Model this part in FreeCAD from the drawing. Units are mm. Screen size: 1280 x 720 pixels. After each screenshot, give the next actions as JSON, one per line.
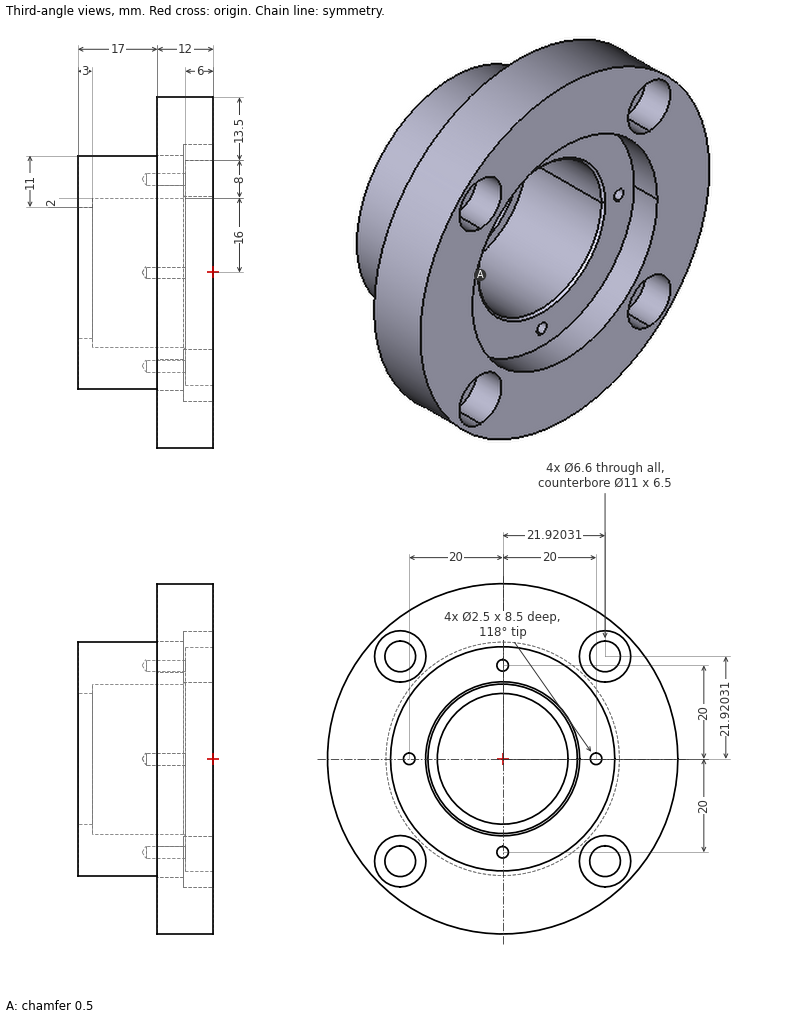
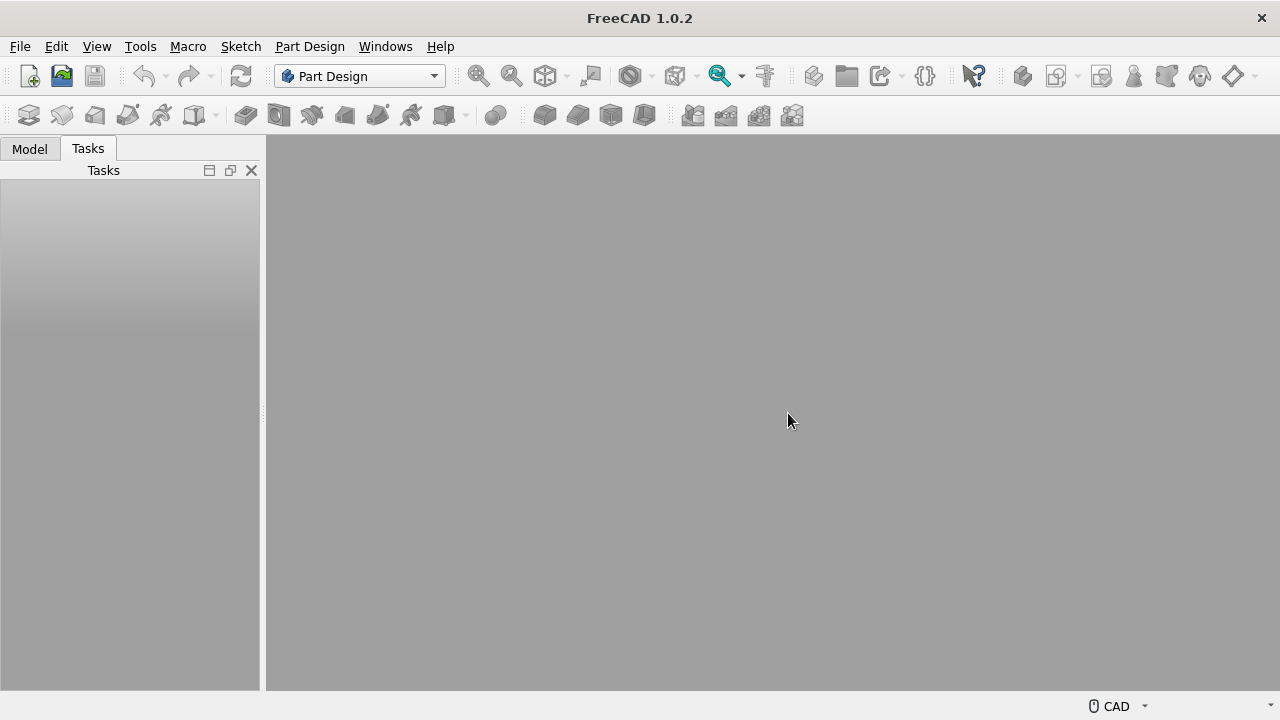
{"action": "key", "text": "ctrl+n"}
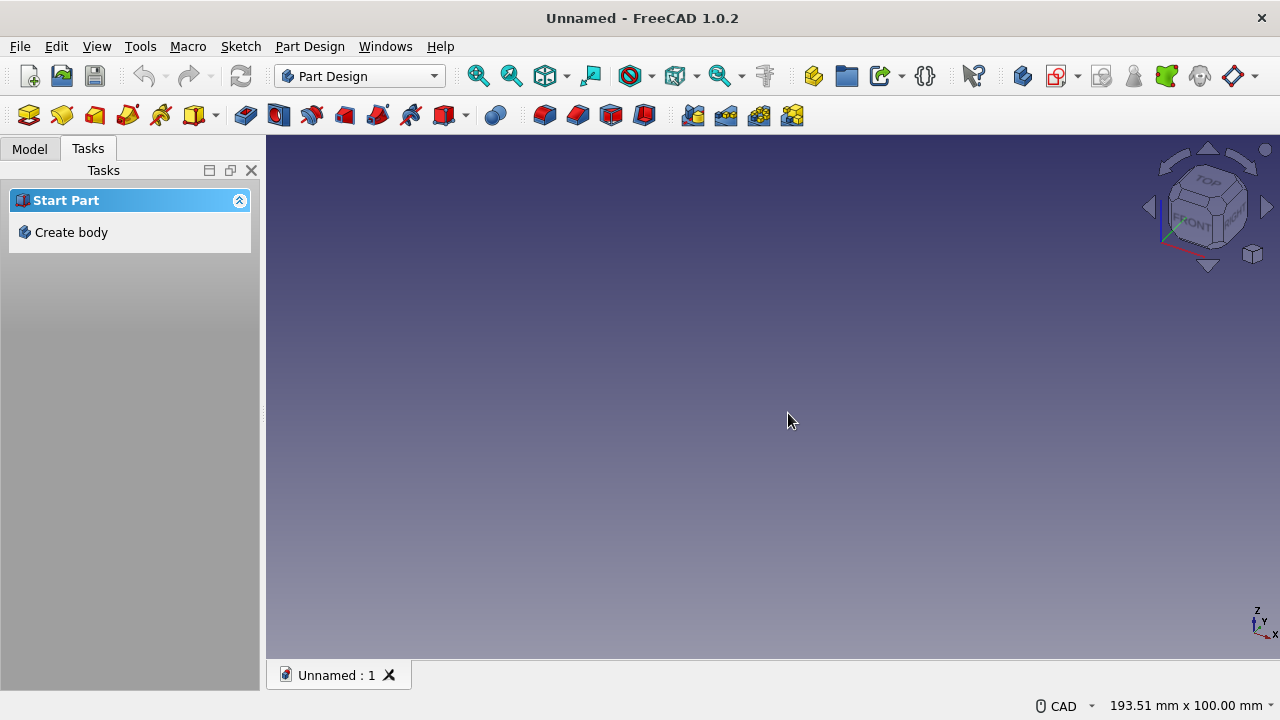
{"action": "left_click", "coordinate": [1056, 76]}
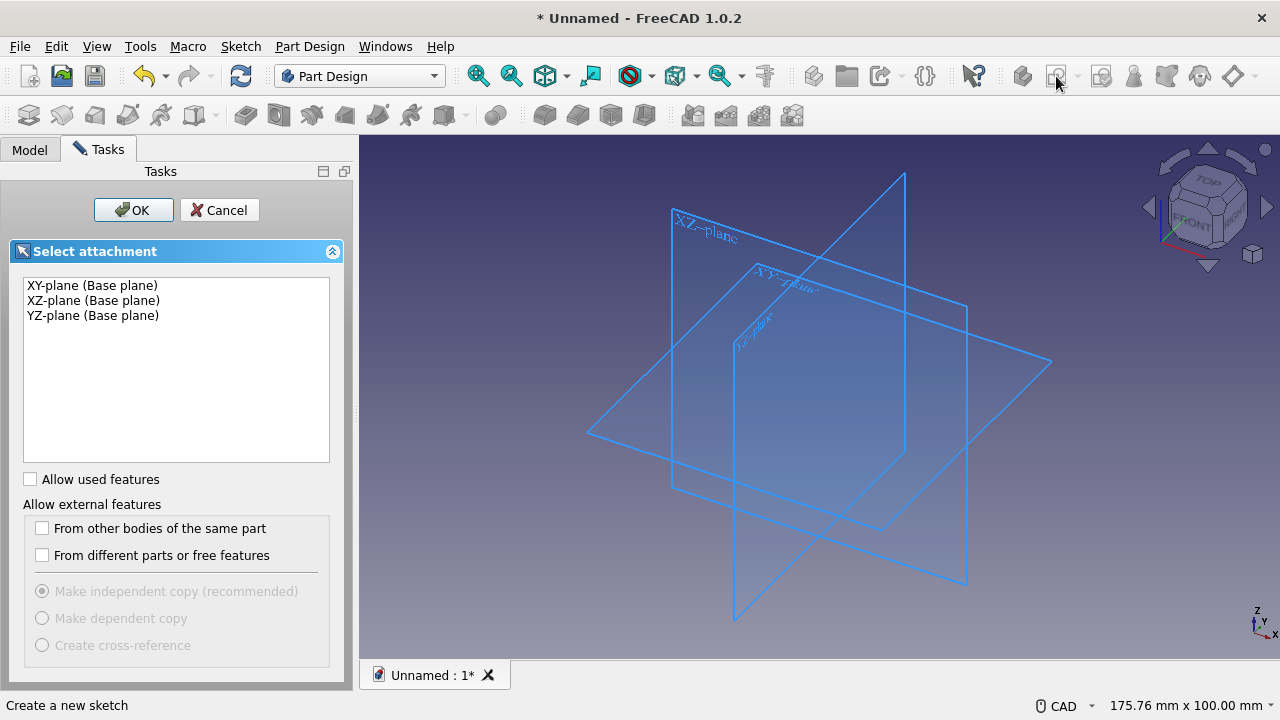
{"action": "left_click", "coordinate": [84, 286]}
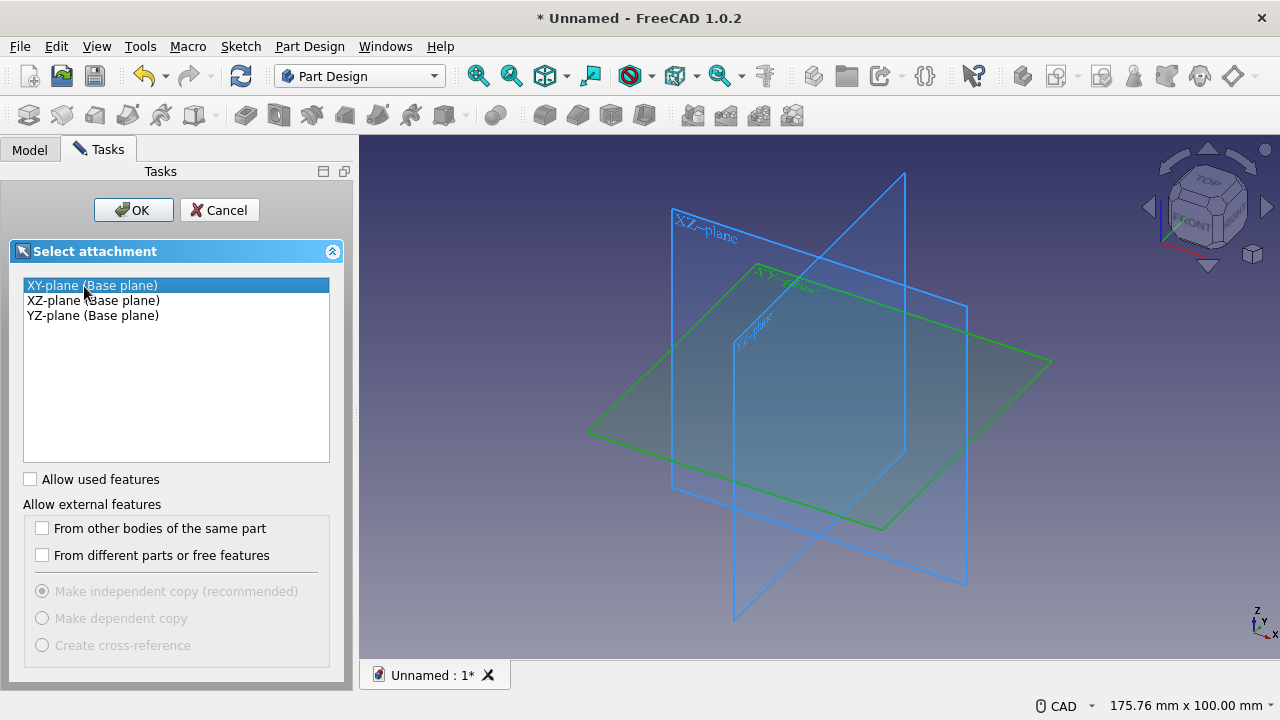
{"action": "left_click", "coordinate": [134, 210]}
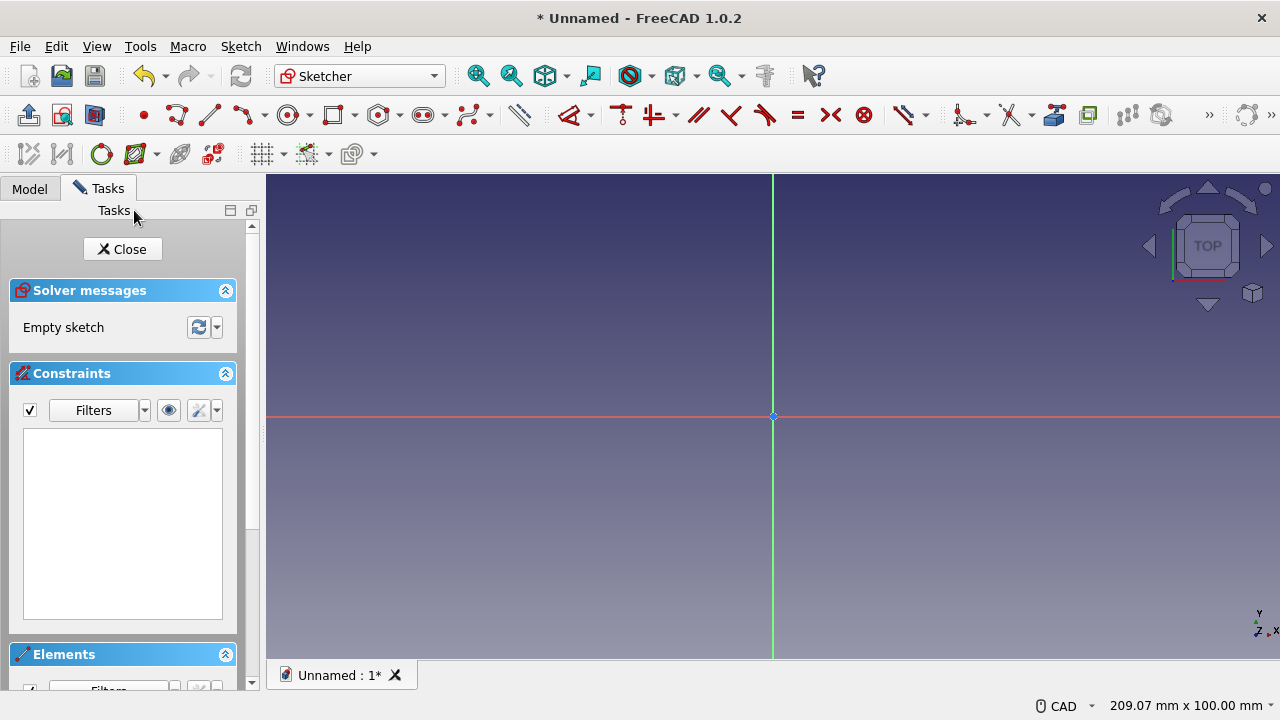
{"action": "scroll", "coordinate": [700, 215], "scroll_direction": "up", "scroll_amount": 3}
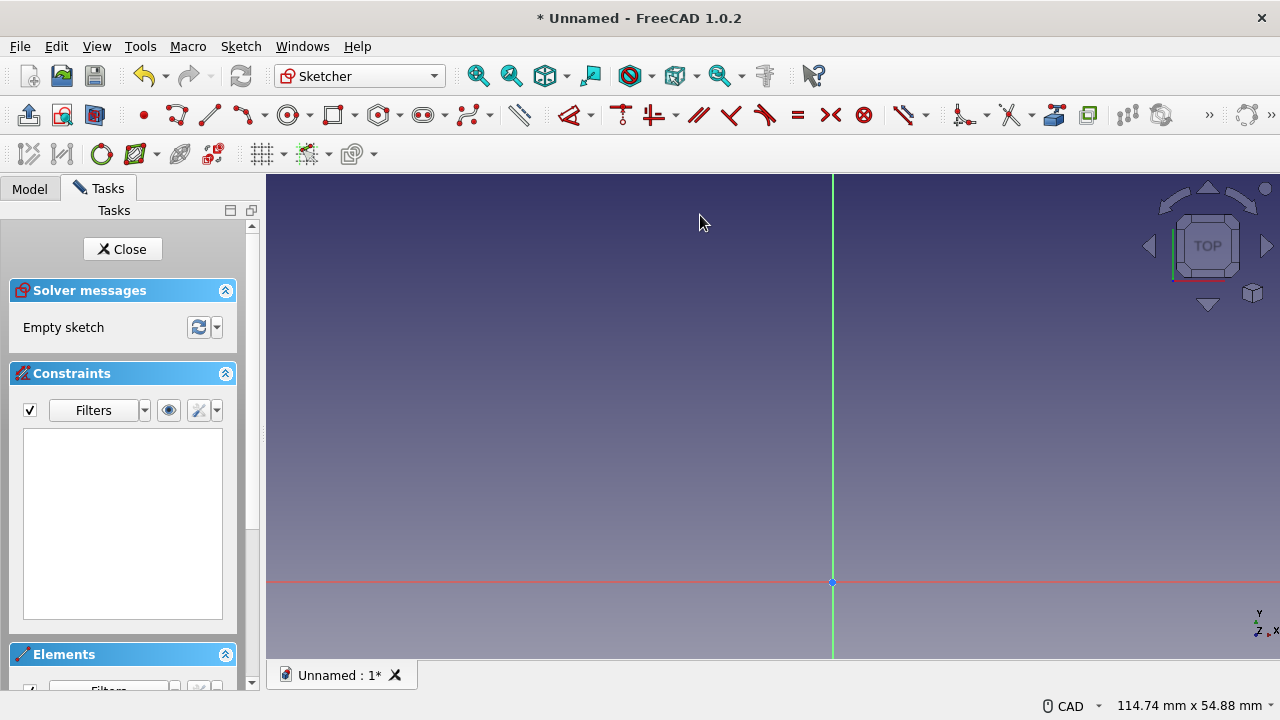
{"action": "key", "text": "g m"}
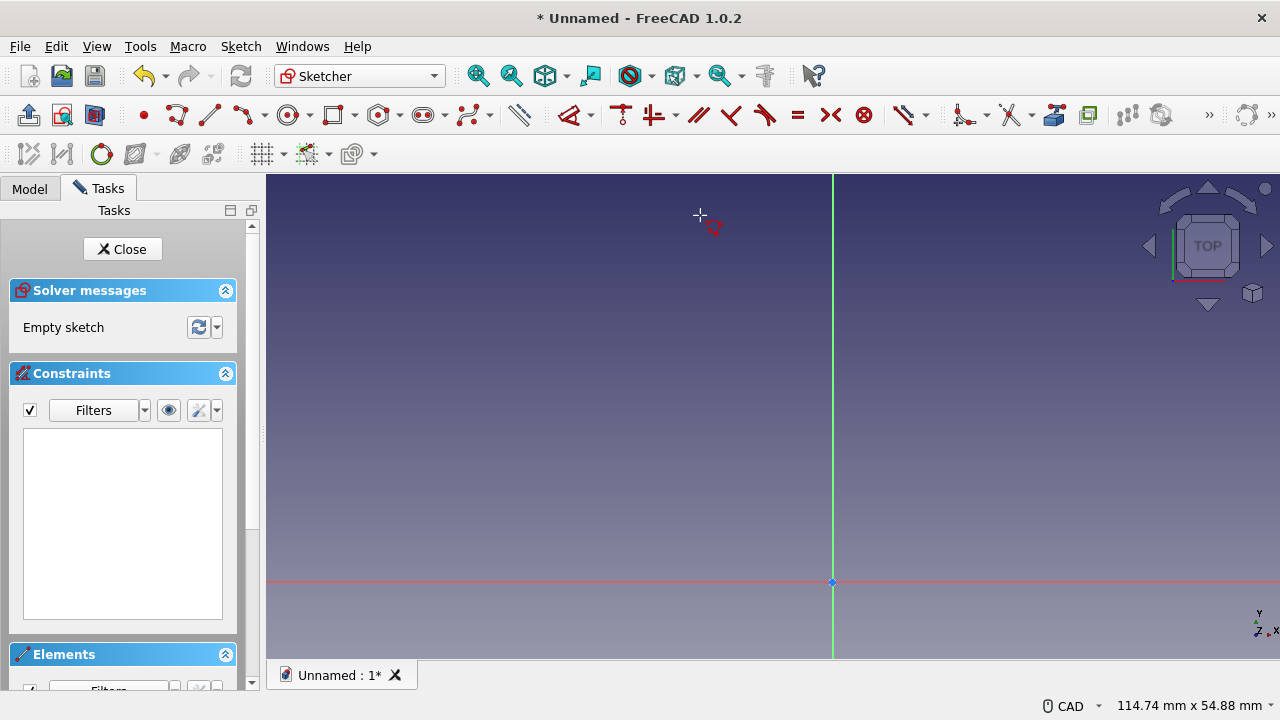
{"action": "left_click", "coordinate": [780, 441]}
{"action": "left_click", "coordinate": [780, 370]}
{"action": "left_click", "coordinate": [833, 370]}
{"action": "left_click", "coordinate": [824, 251]}
{"action": "left_click", "coordinate": [727, 251]}
{"action": "left_click", "coordinate": [727, 361]}
{"action": "left_click", "coordinate": [576, 361]}
{"action": "left_click", "coordinate": [576, 458]}
{"action": "left_click", "coordinate": [603, 458]}
{"action": "left_click", "coordinate": [603, 441]}
{"action": "left_click", "coordinate": [780, 442]}
{"action": "key", "text": "Escape"}
{"action": "key", "text": "Escape"}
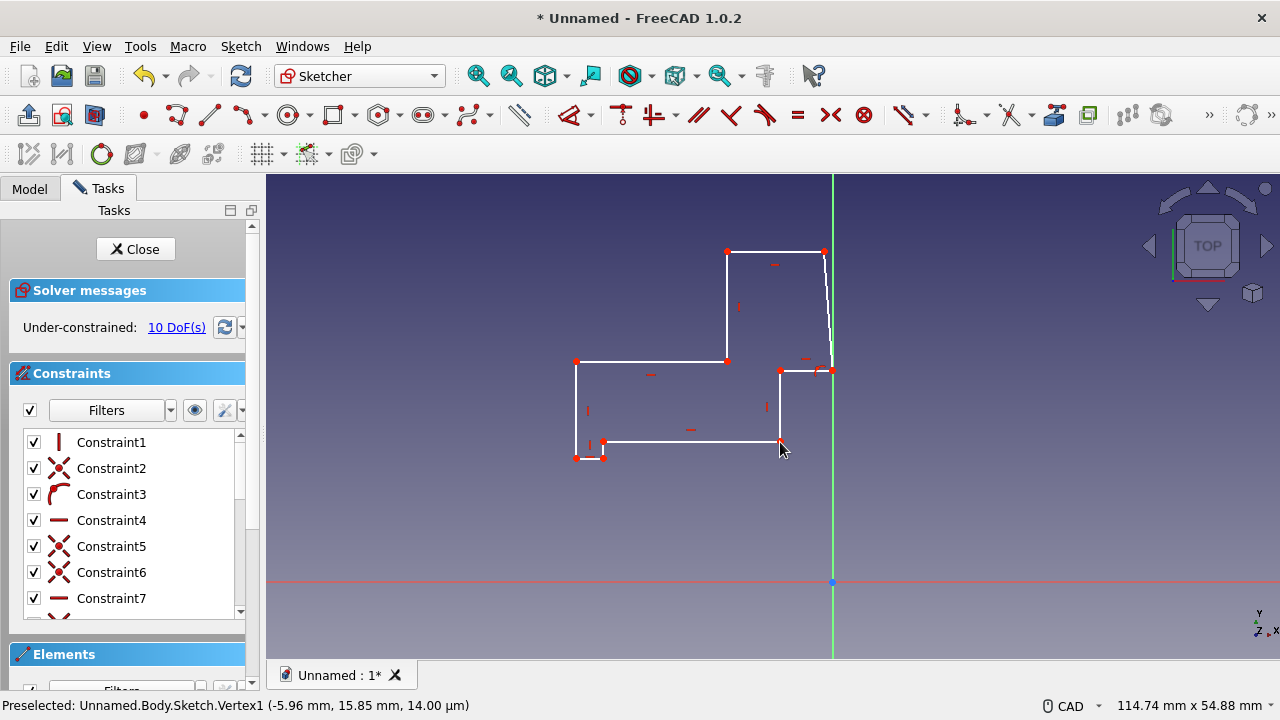
{"action": "left_click", "coordinate": [830, 335]}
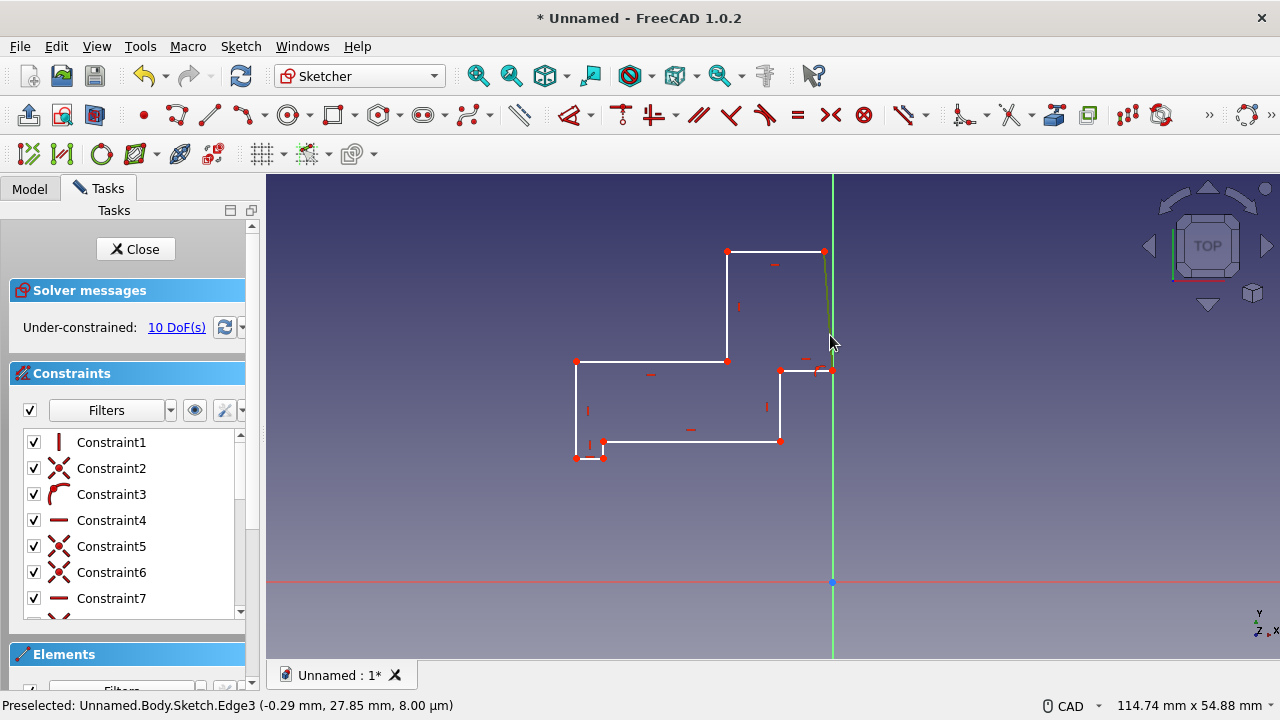
{"action": "key", "text": "v"}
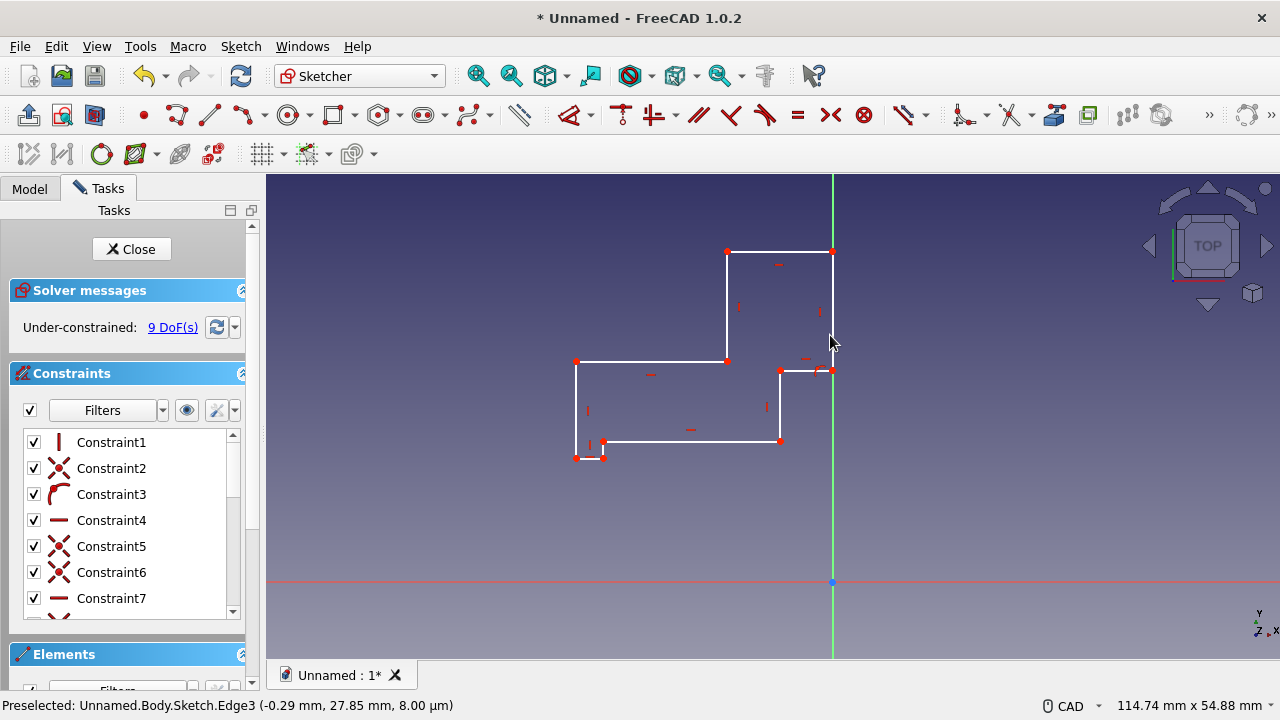
{"action": "left_click", "coordinate": [780, 421]}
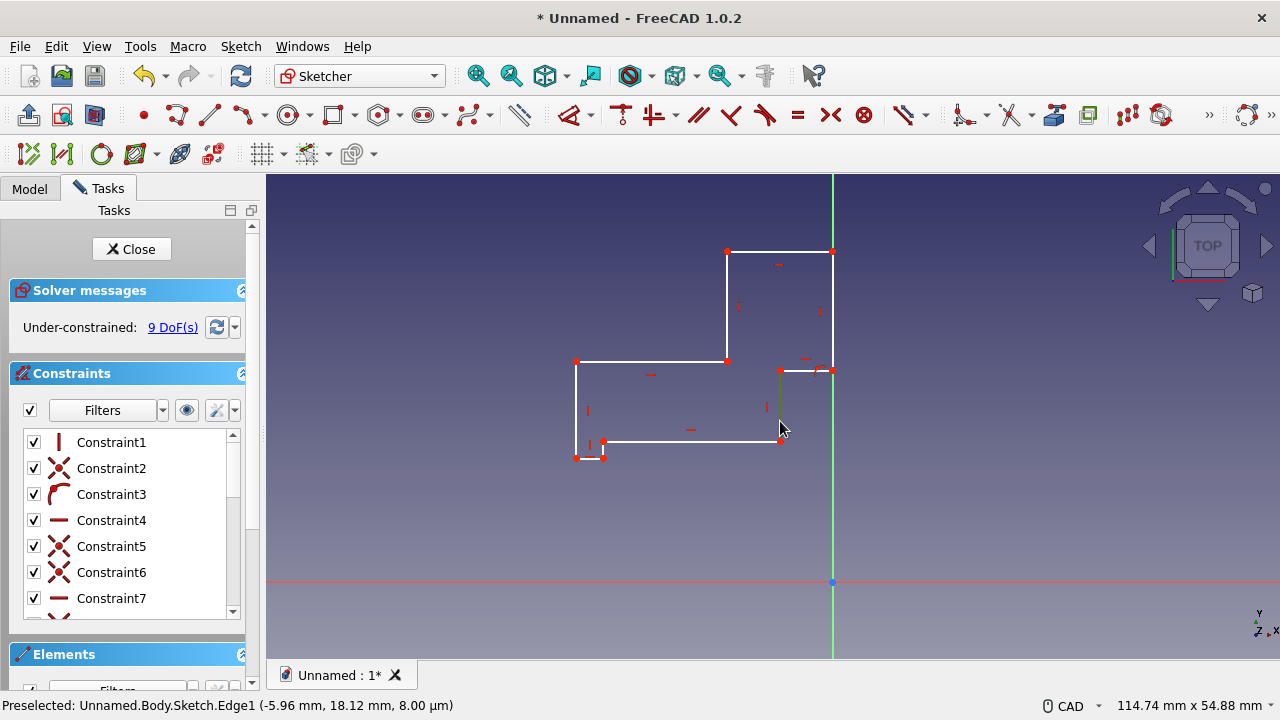
{"action": "key", "text": "i"}